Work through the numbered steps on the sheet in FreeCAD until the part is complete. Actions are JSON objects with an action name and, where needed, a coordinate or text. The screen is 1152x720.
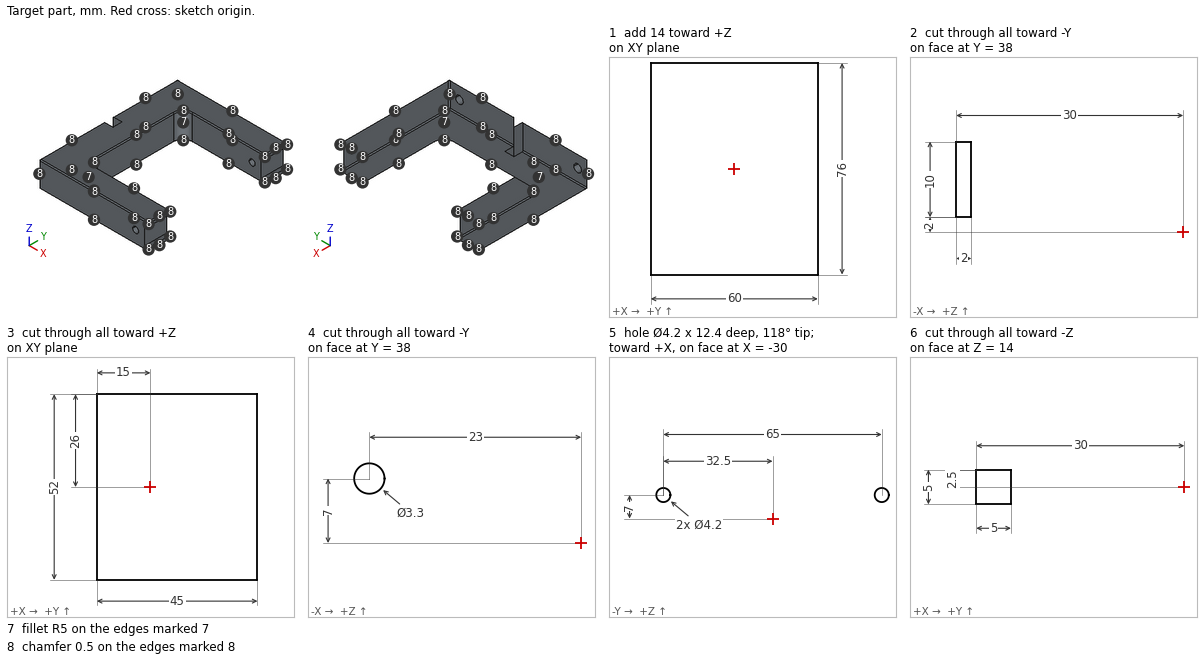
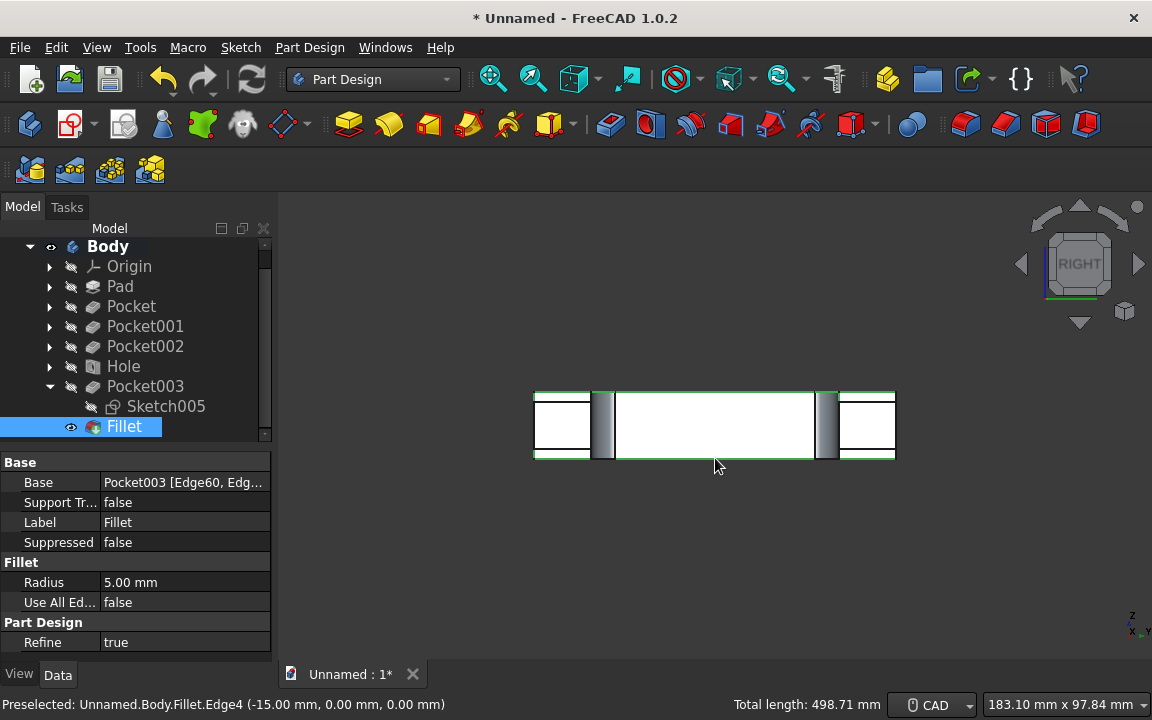
{"action": "left_click", "coordinate": [832, 458], "text": "ctrl"}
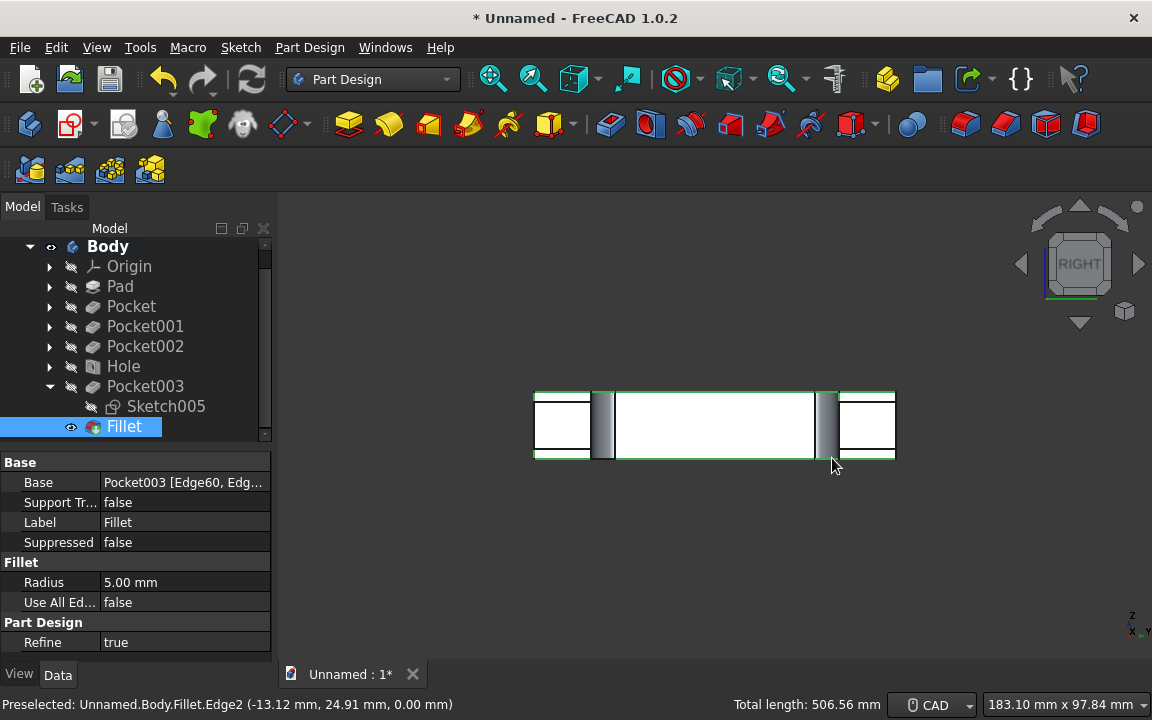
{"action": "left_click", "coordinate": [598, 458], "text": "ctrl"}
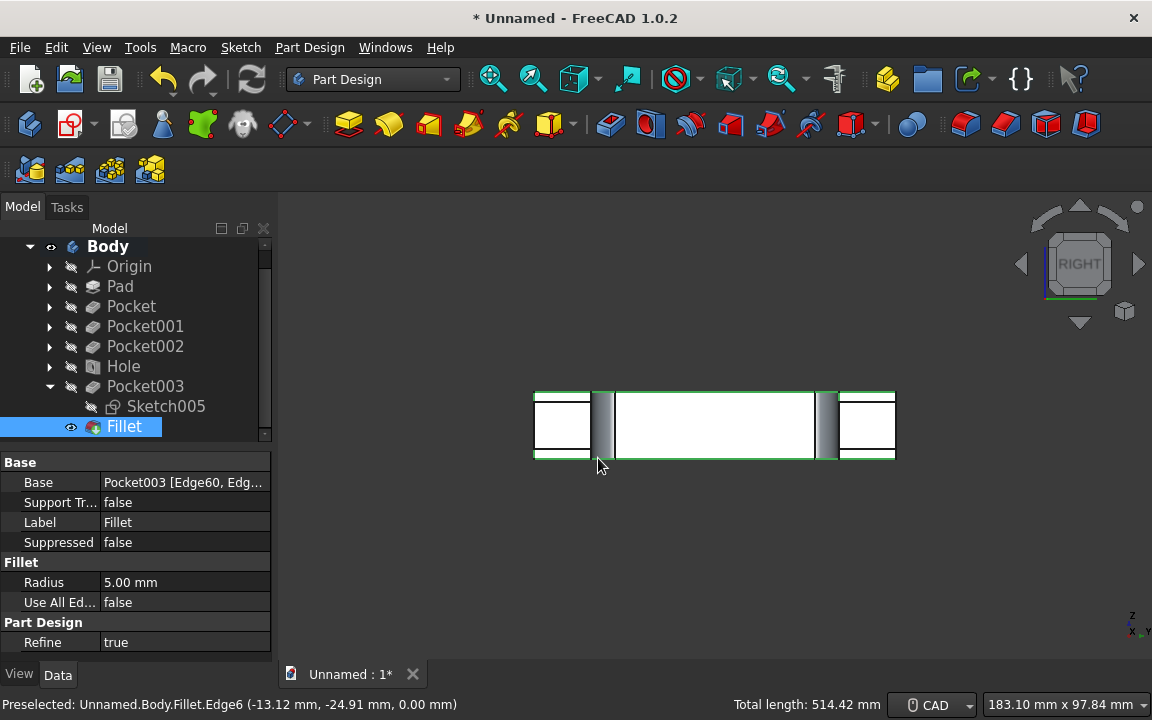
{"action": "scroll", "coordinate": [896, 453], "scroll_direction": "up", "scroll_amount": 8}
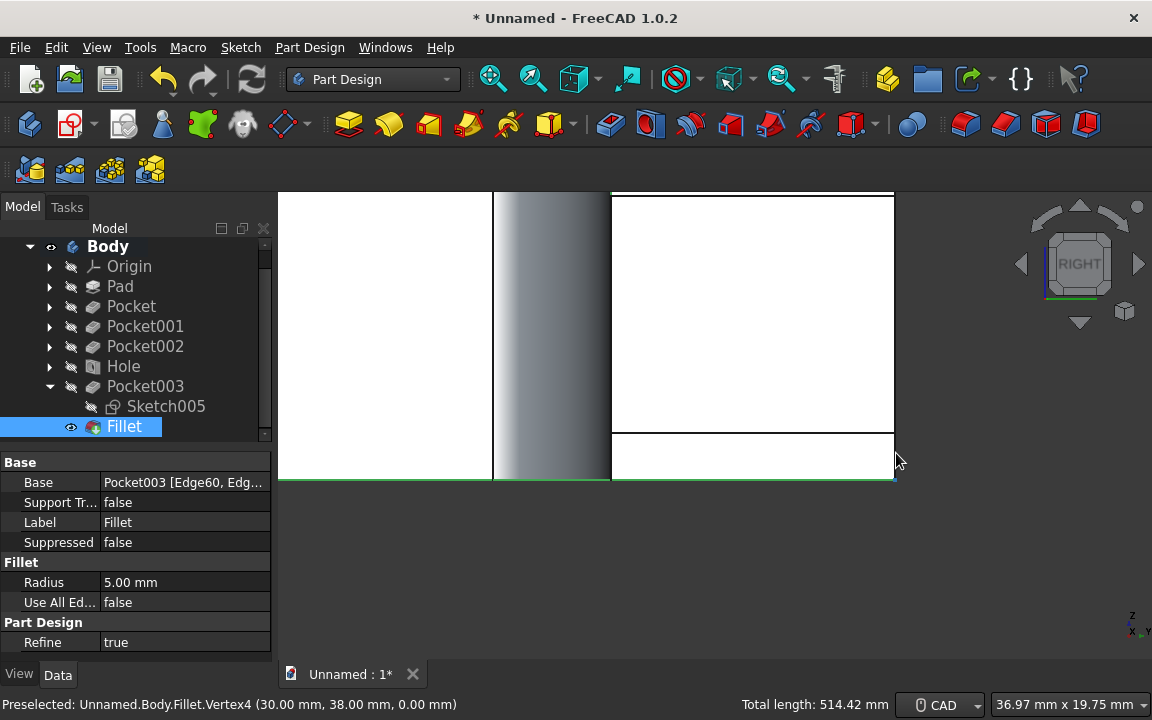
{"action": "left_click", "coordinate": [895, 455], "text": "ctrl"}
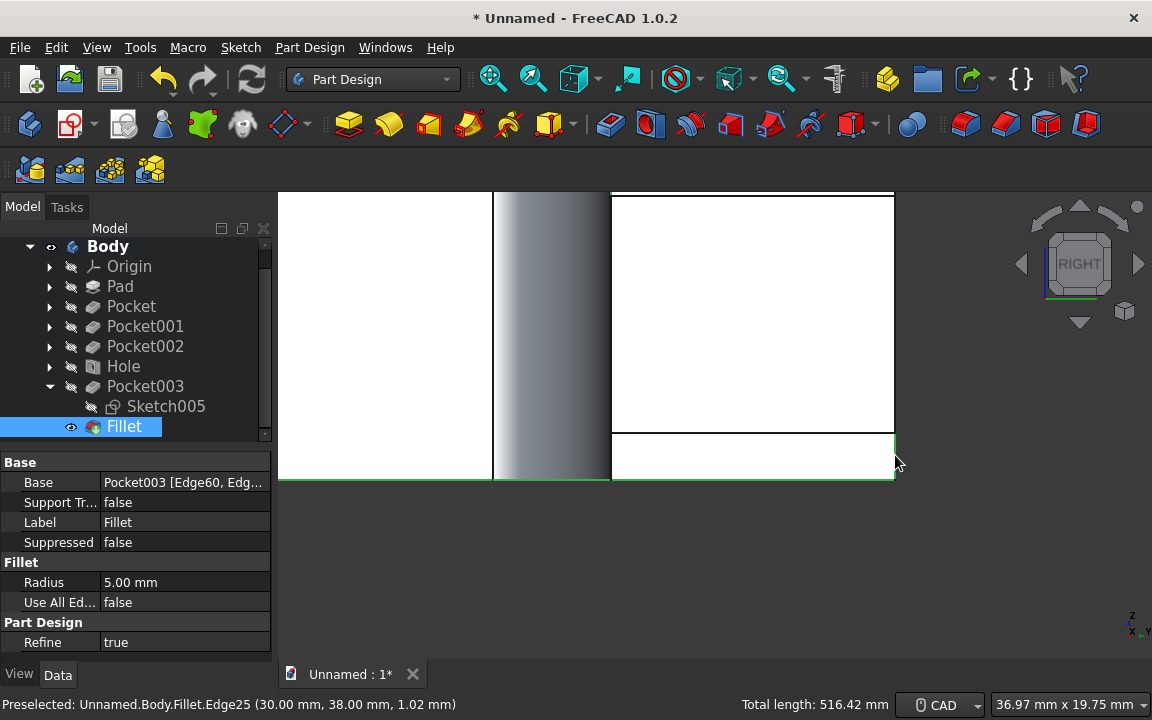
{"action": "left_click", "coordinate": [611, 455], "text": "ctrl"}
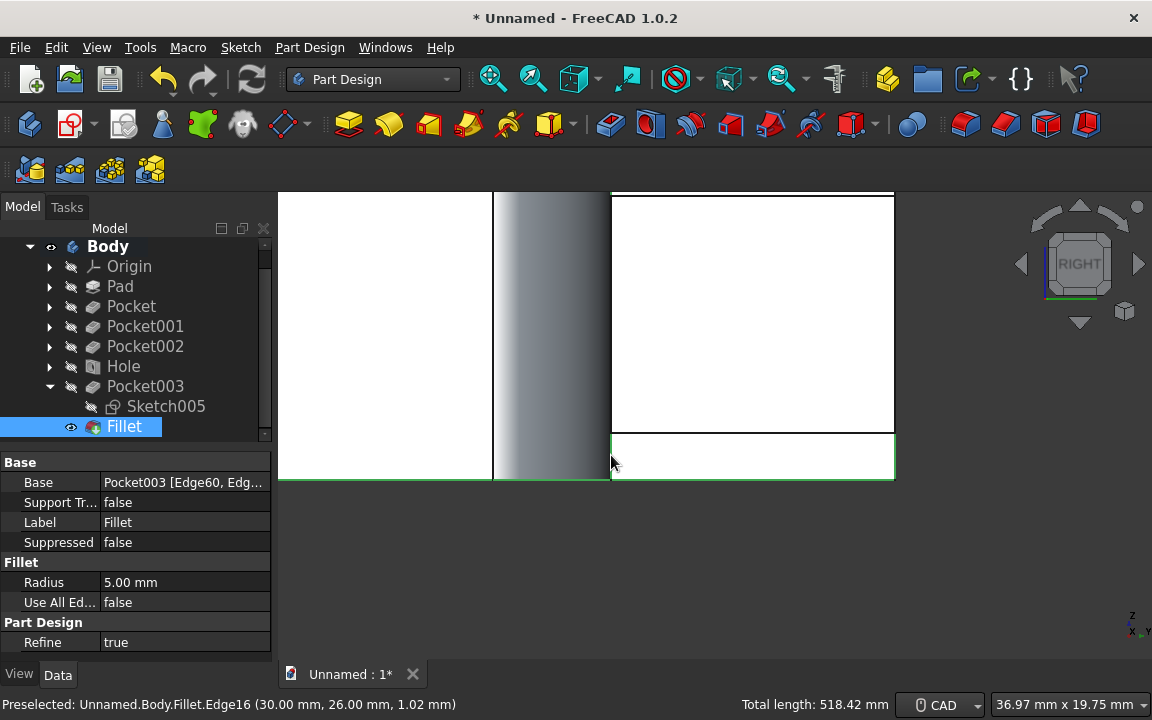
{"action": "key", "text": "v f"}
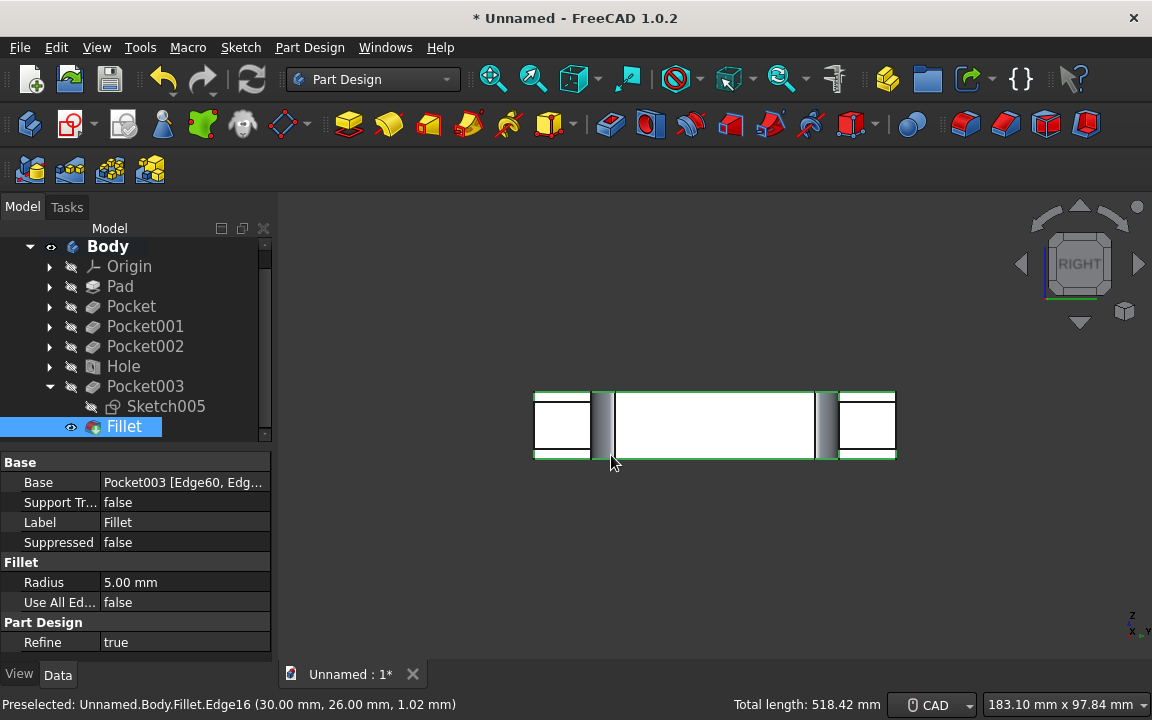
{"action": "key", "text": "5"}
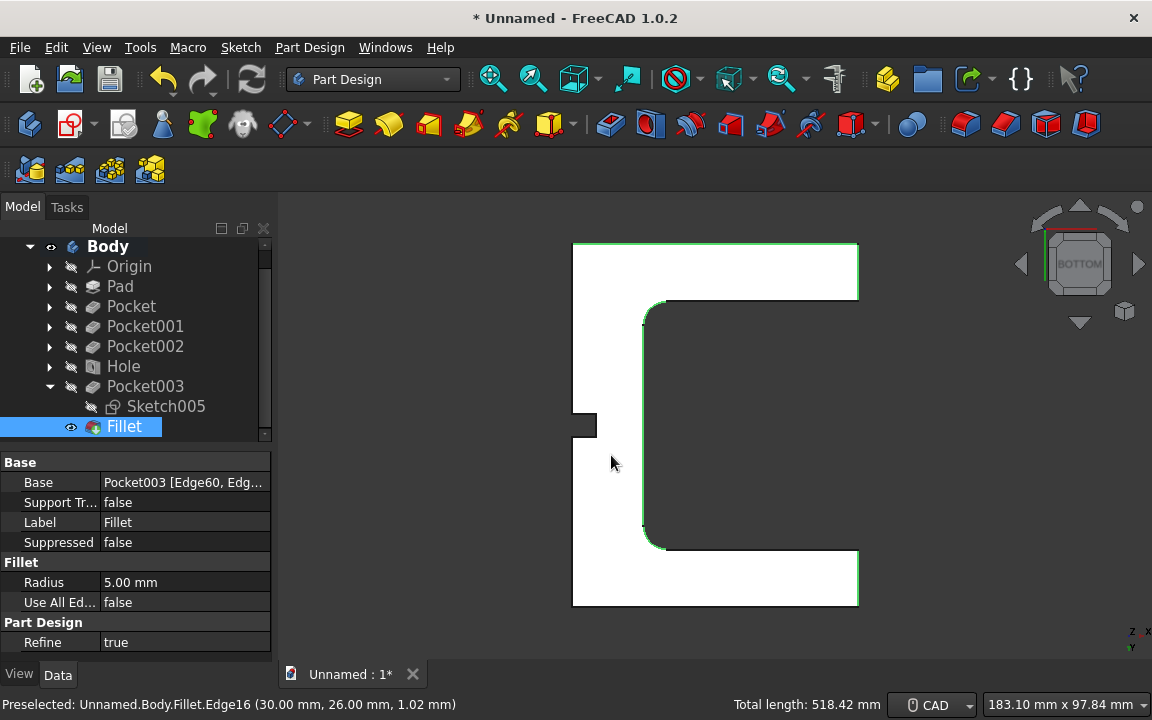
{"action": "left_click", "coordinate": [763, 300], "text": "ctrl"}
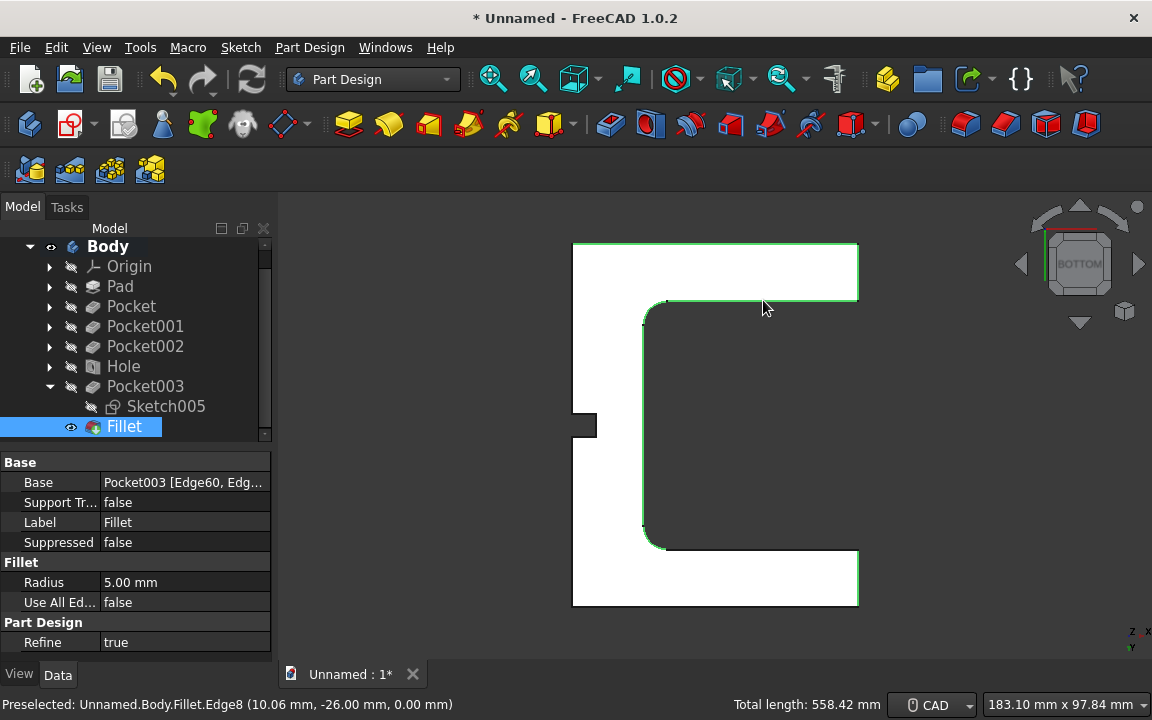
{"action": "left_click", "coordinate": [572, 521], "text": "ctrl"}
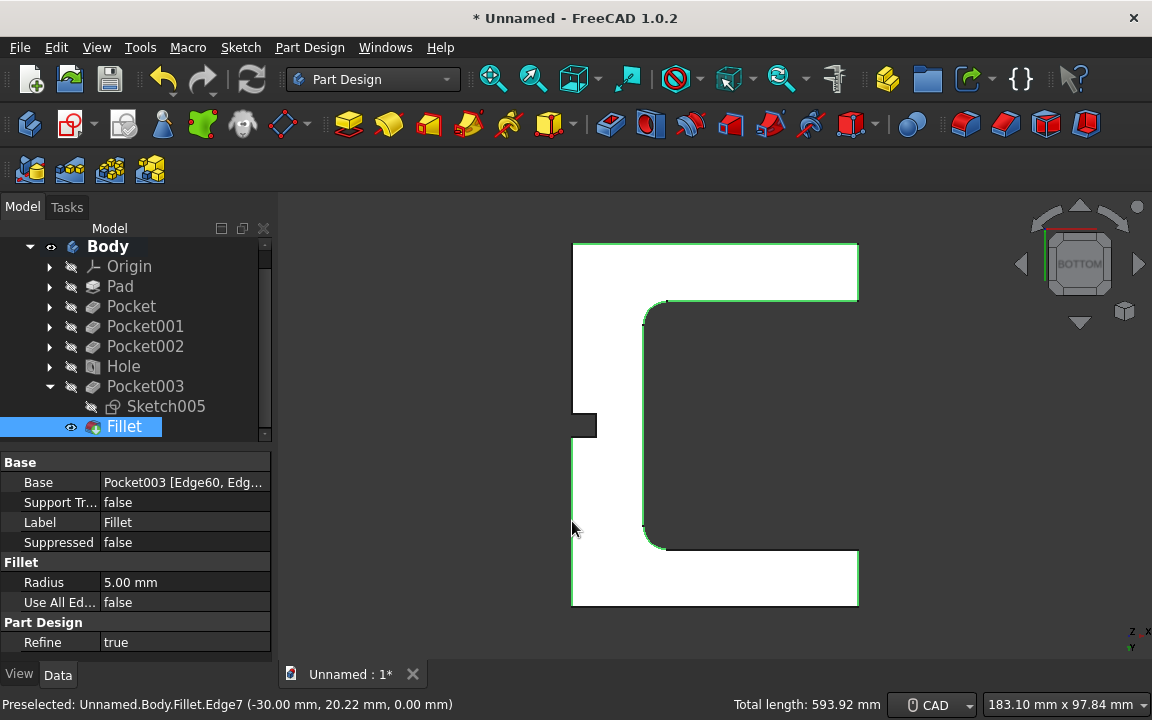
{"action": "left_click", "coordinate": [715, 606], "text": "ctrl"}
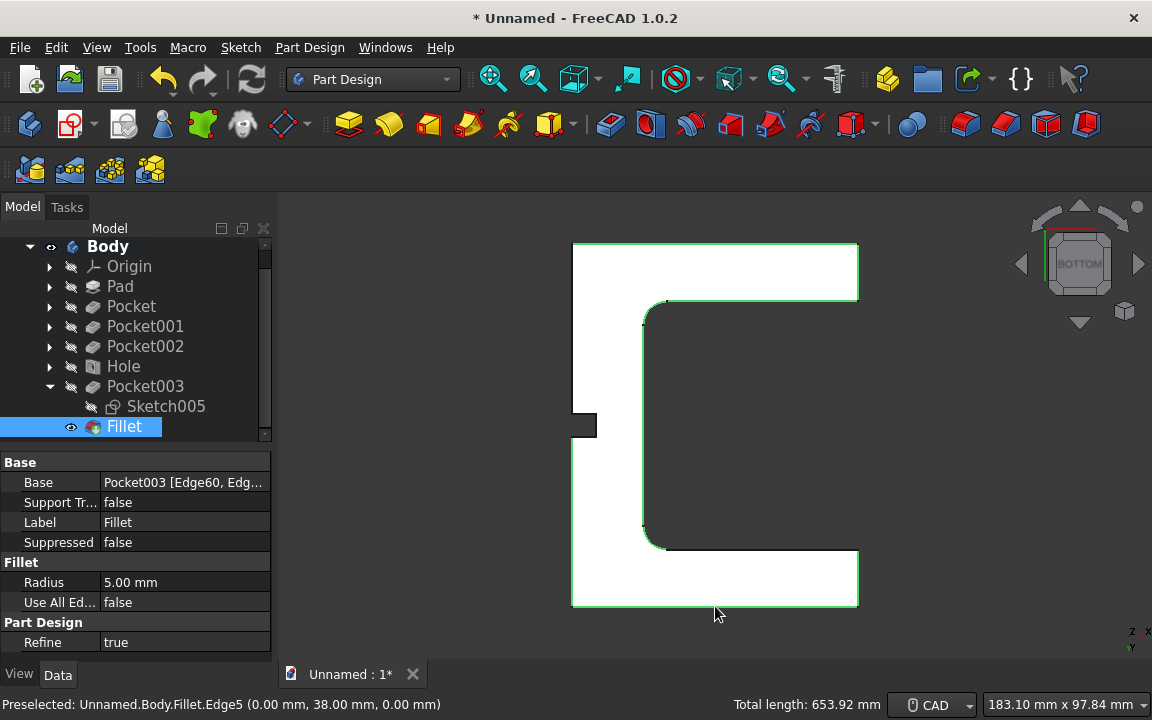
{"action": "left_click", "coordinate": [572, 328], "text": "ctrl"}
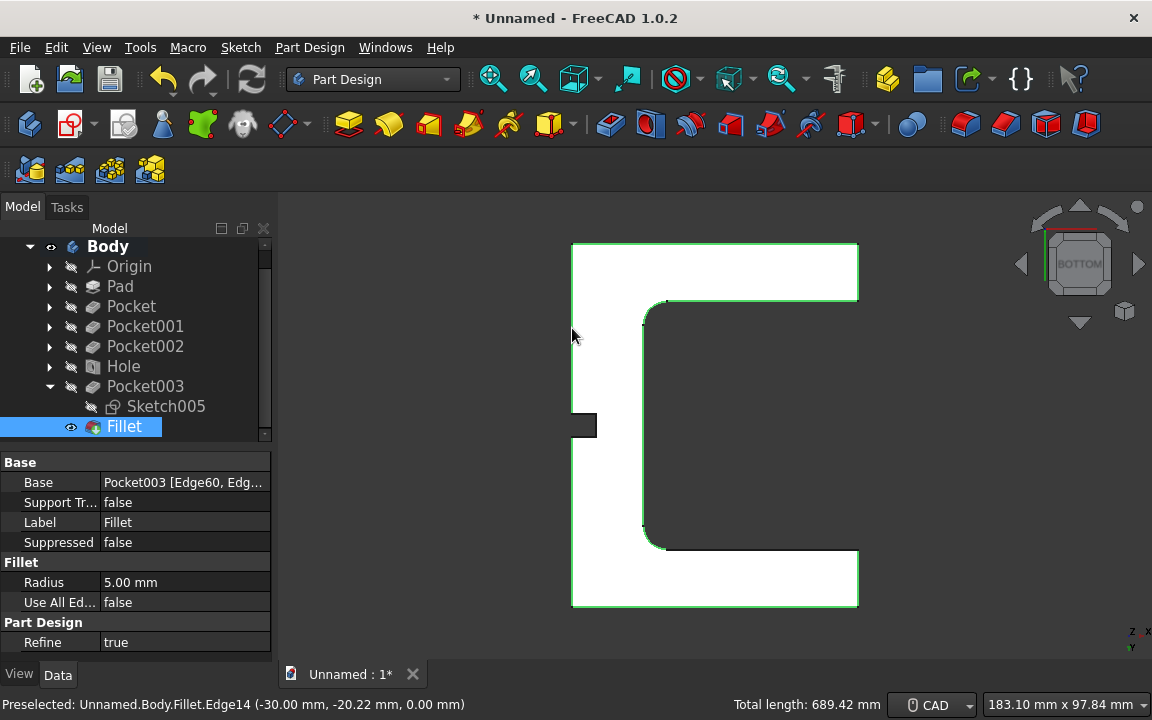
{"action": "left_click", "coordinate": [763, 549], "text": "ctrl"}